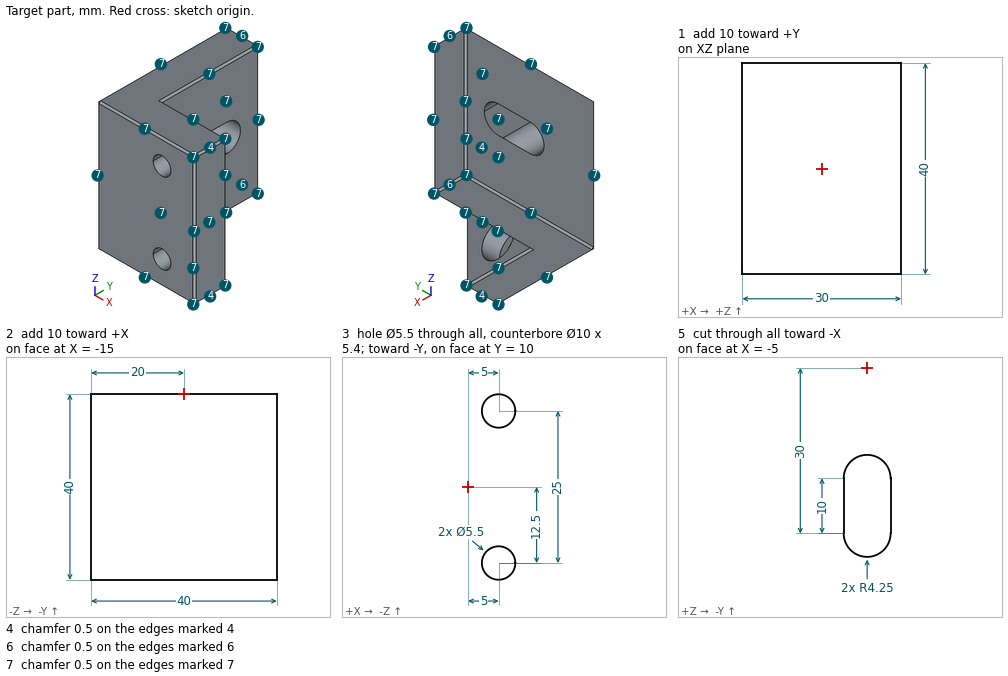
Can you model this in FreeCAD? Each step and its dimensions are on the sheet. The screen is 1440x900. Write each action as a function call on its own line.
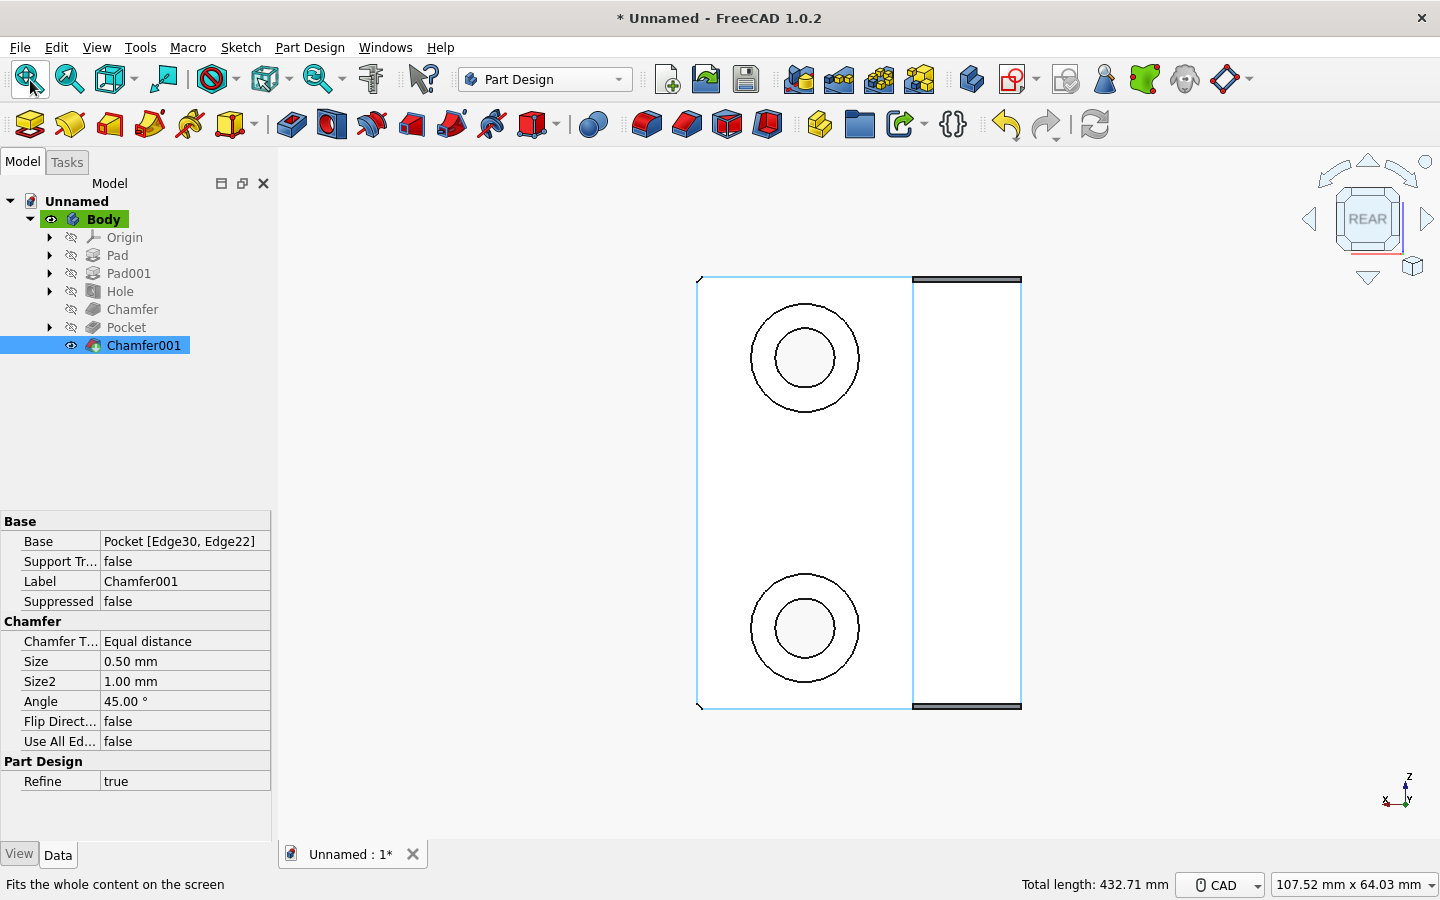
scroll(700, 279, up, 9)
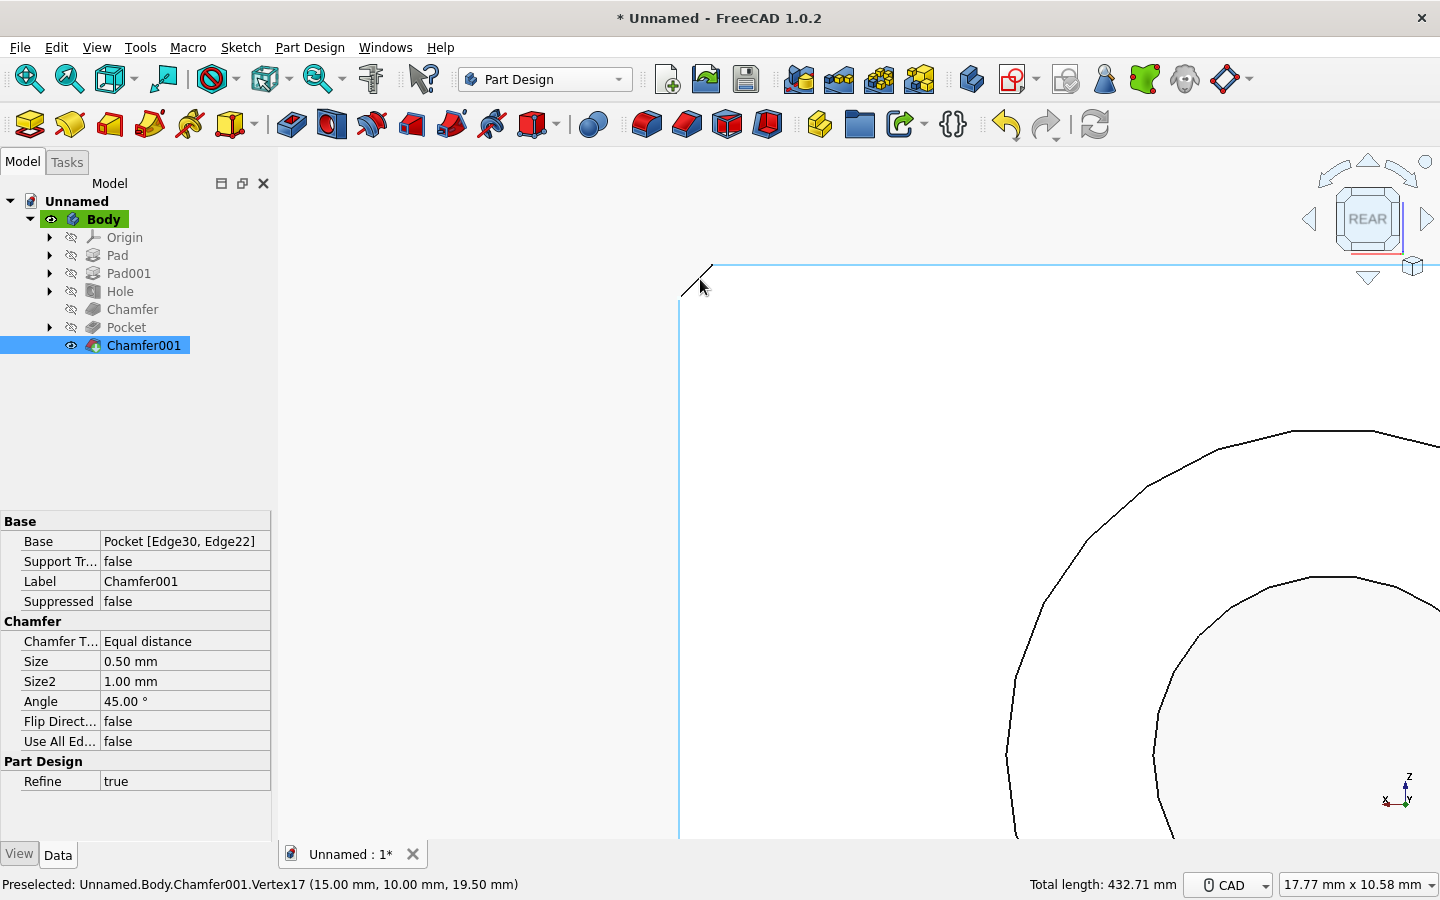
click(30, 80)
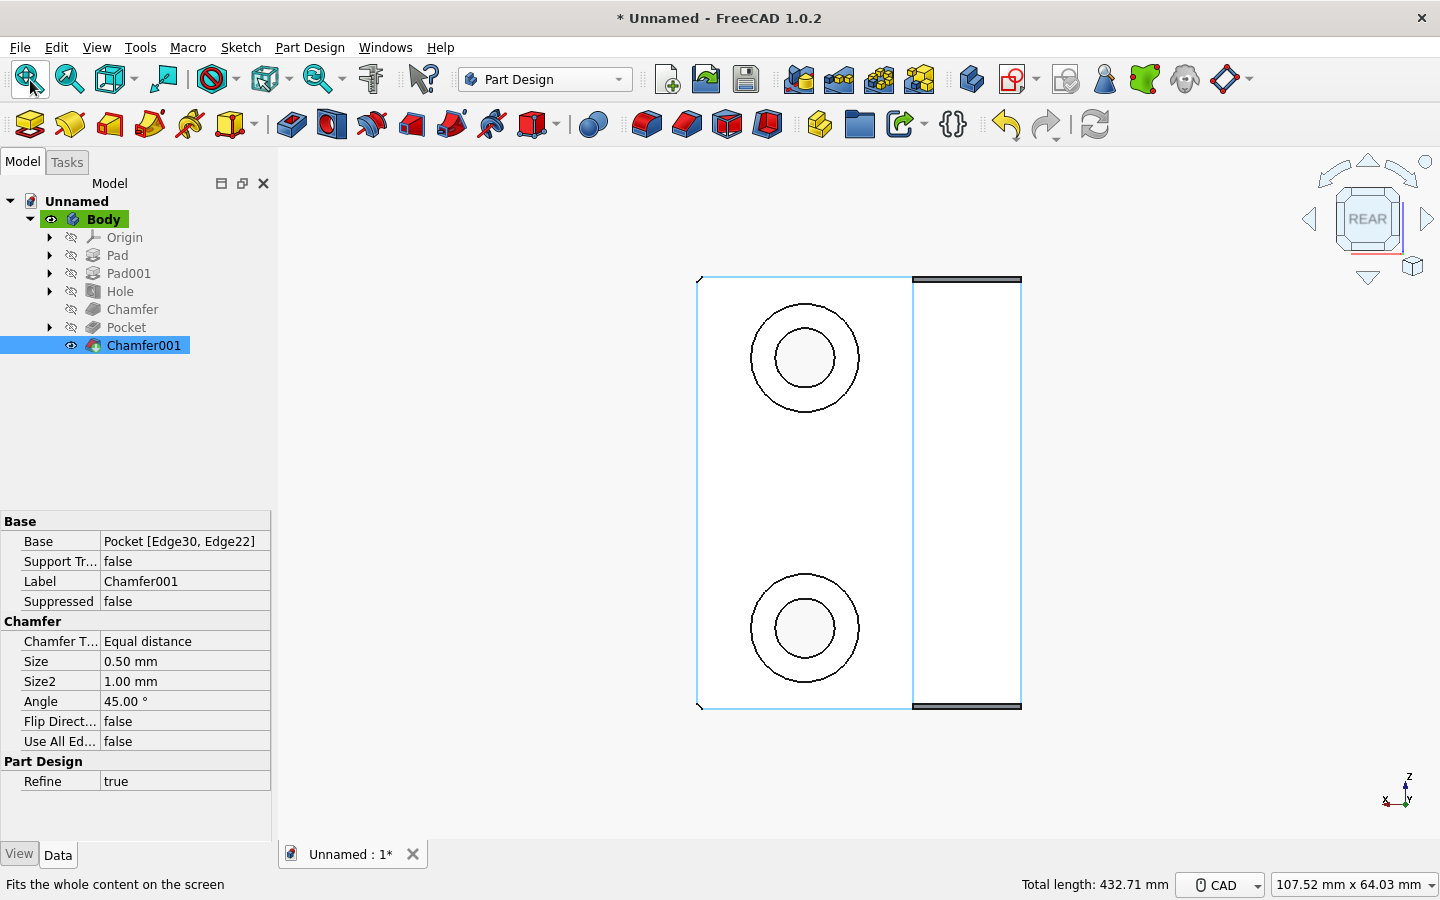
key(6)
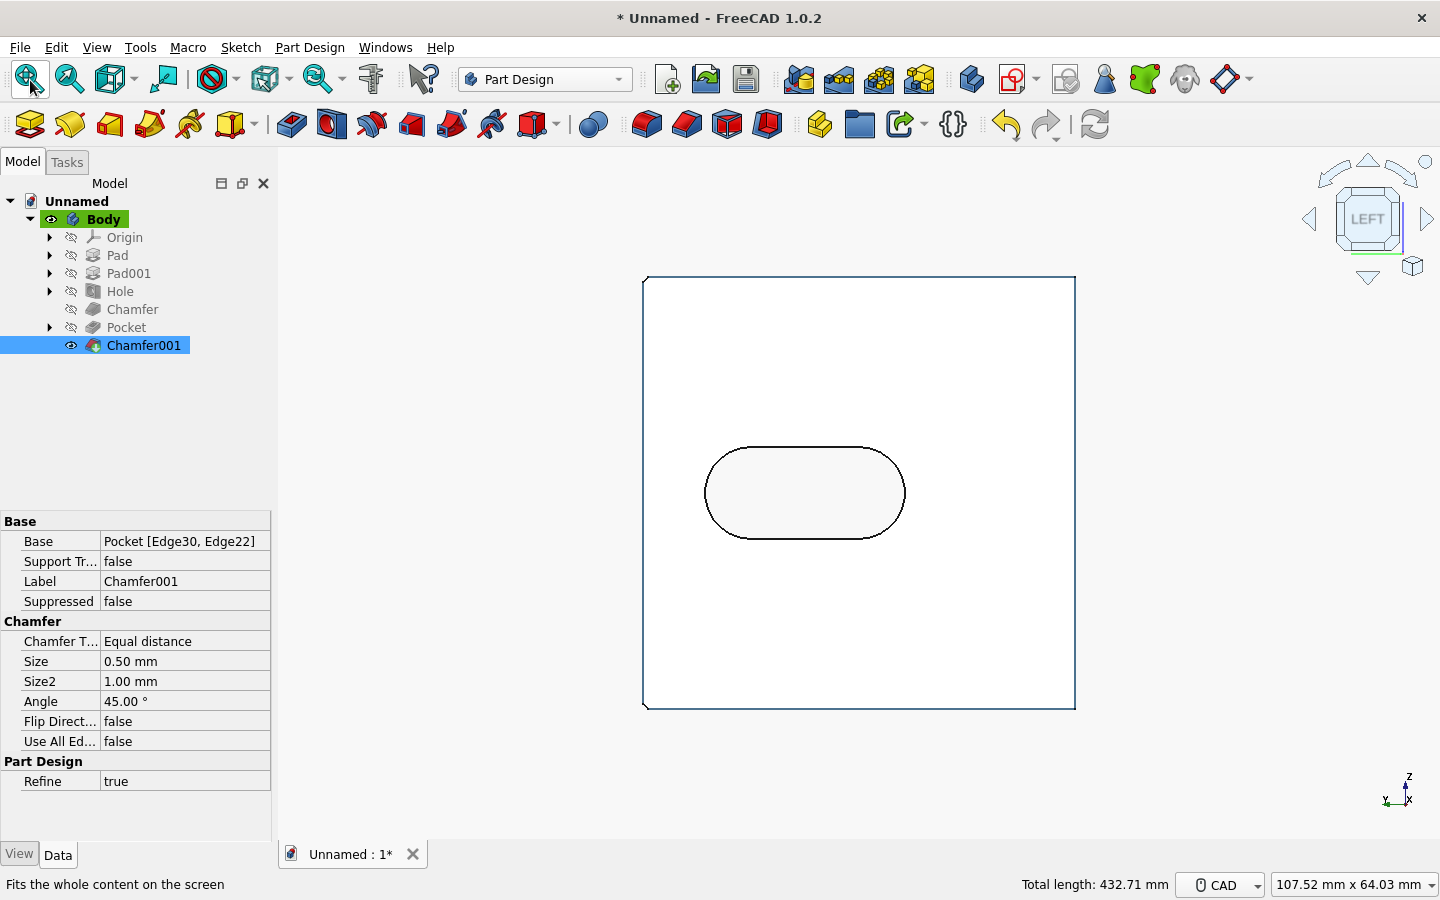
scroll(1075, 279, up, 9)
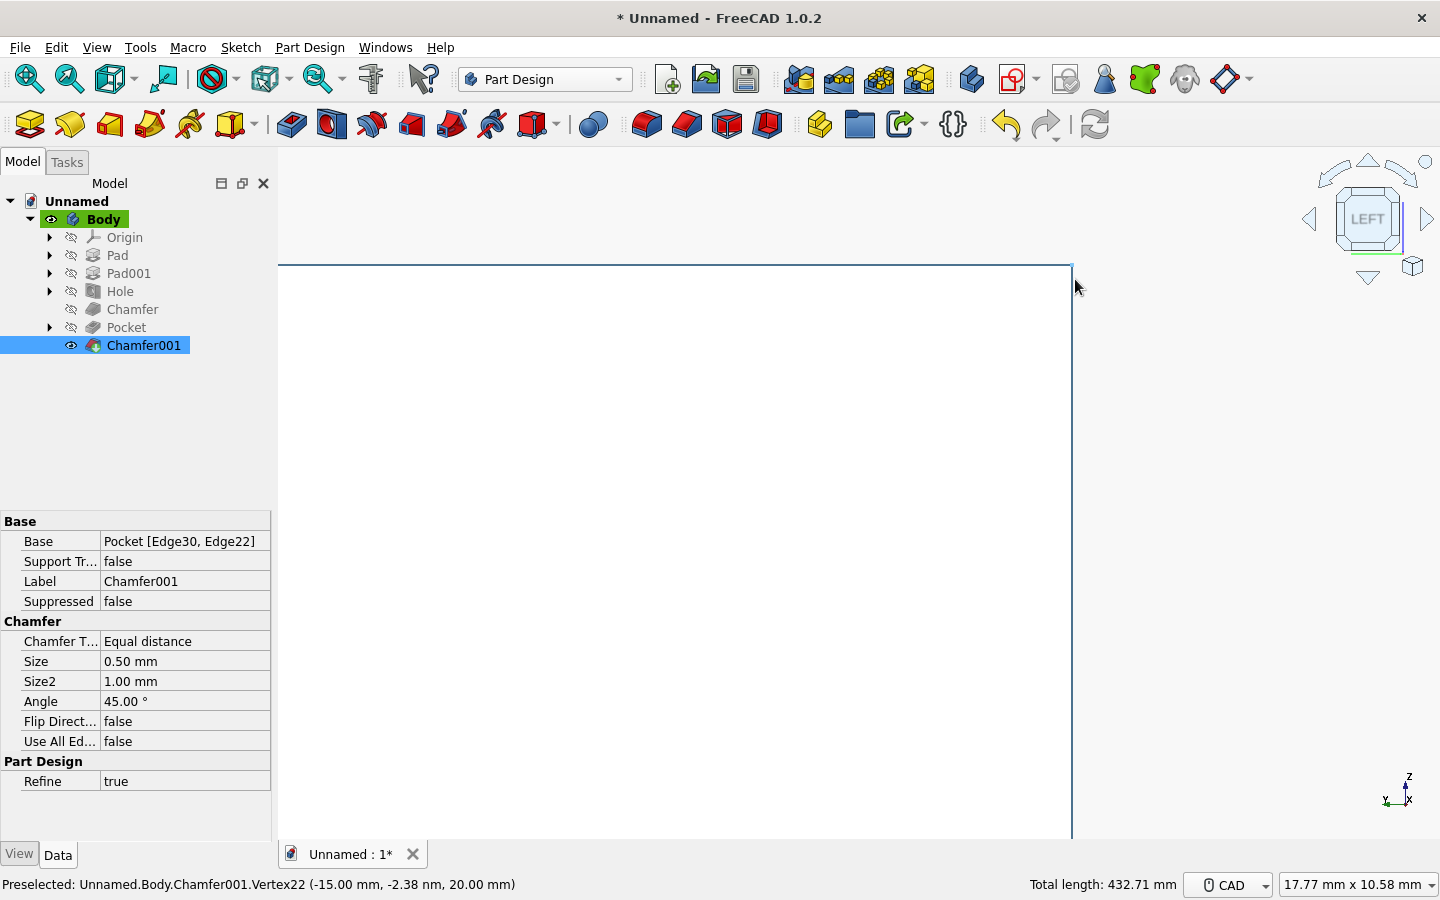
click(30, 80)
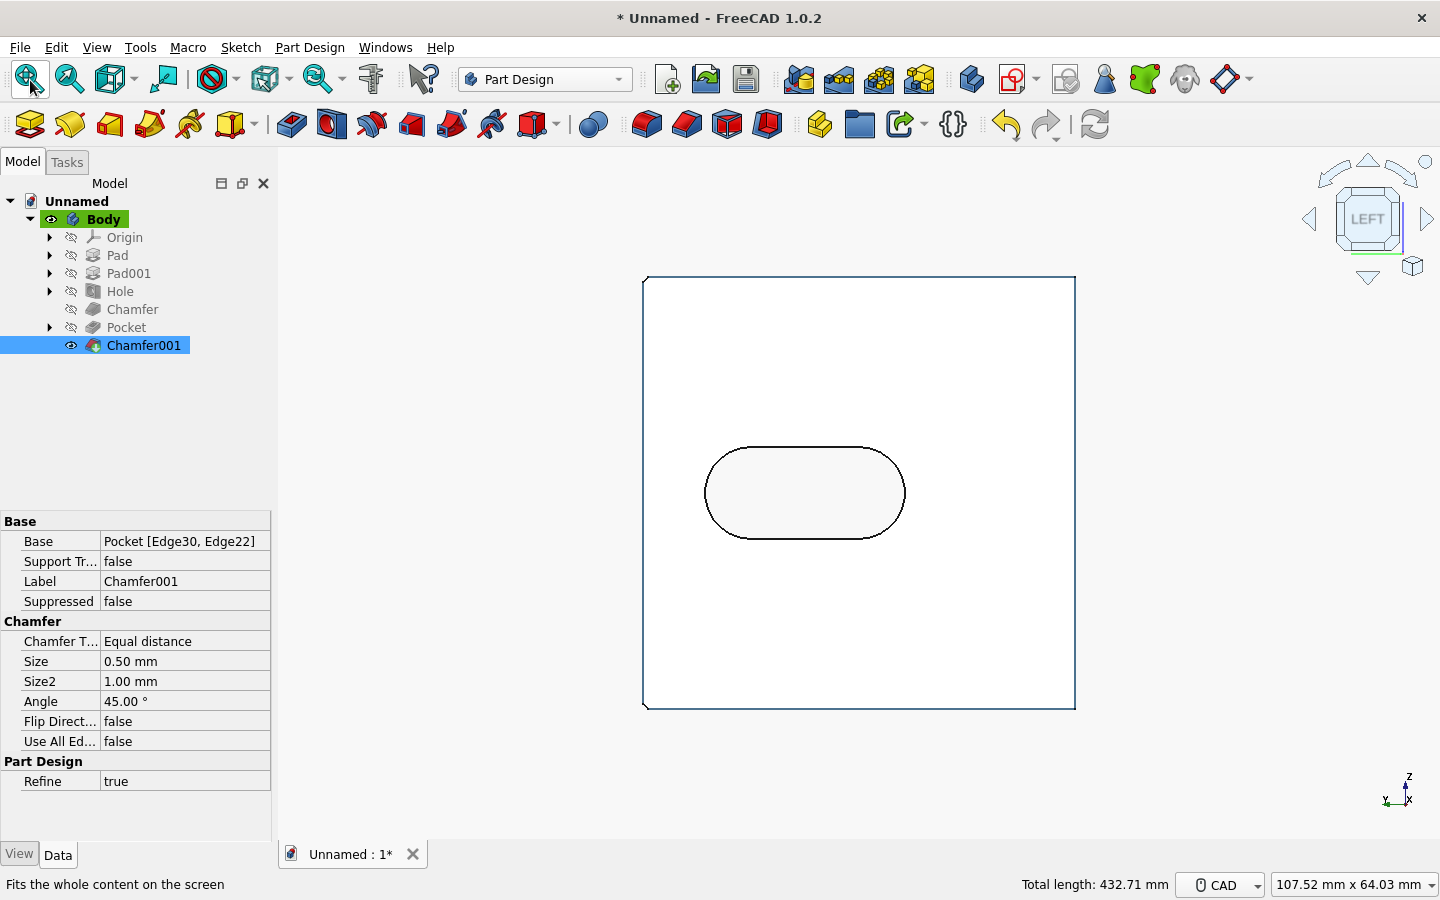
key(v)
key(3)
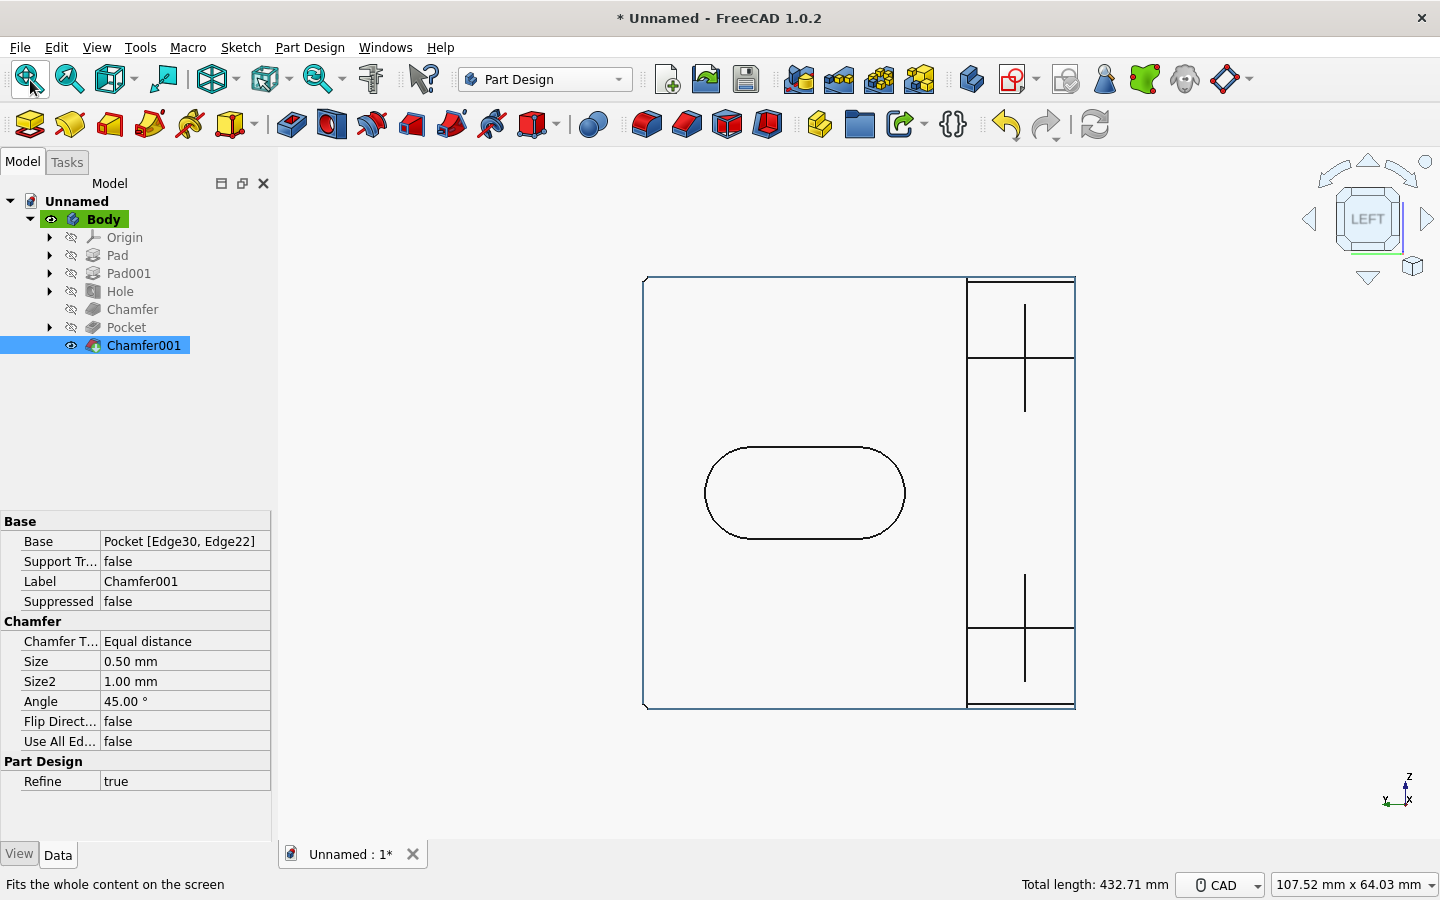
key(0)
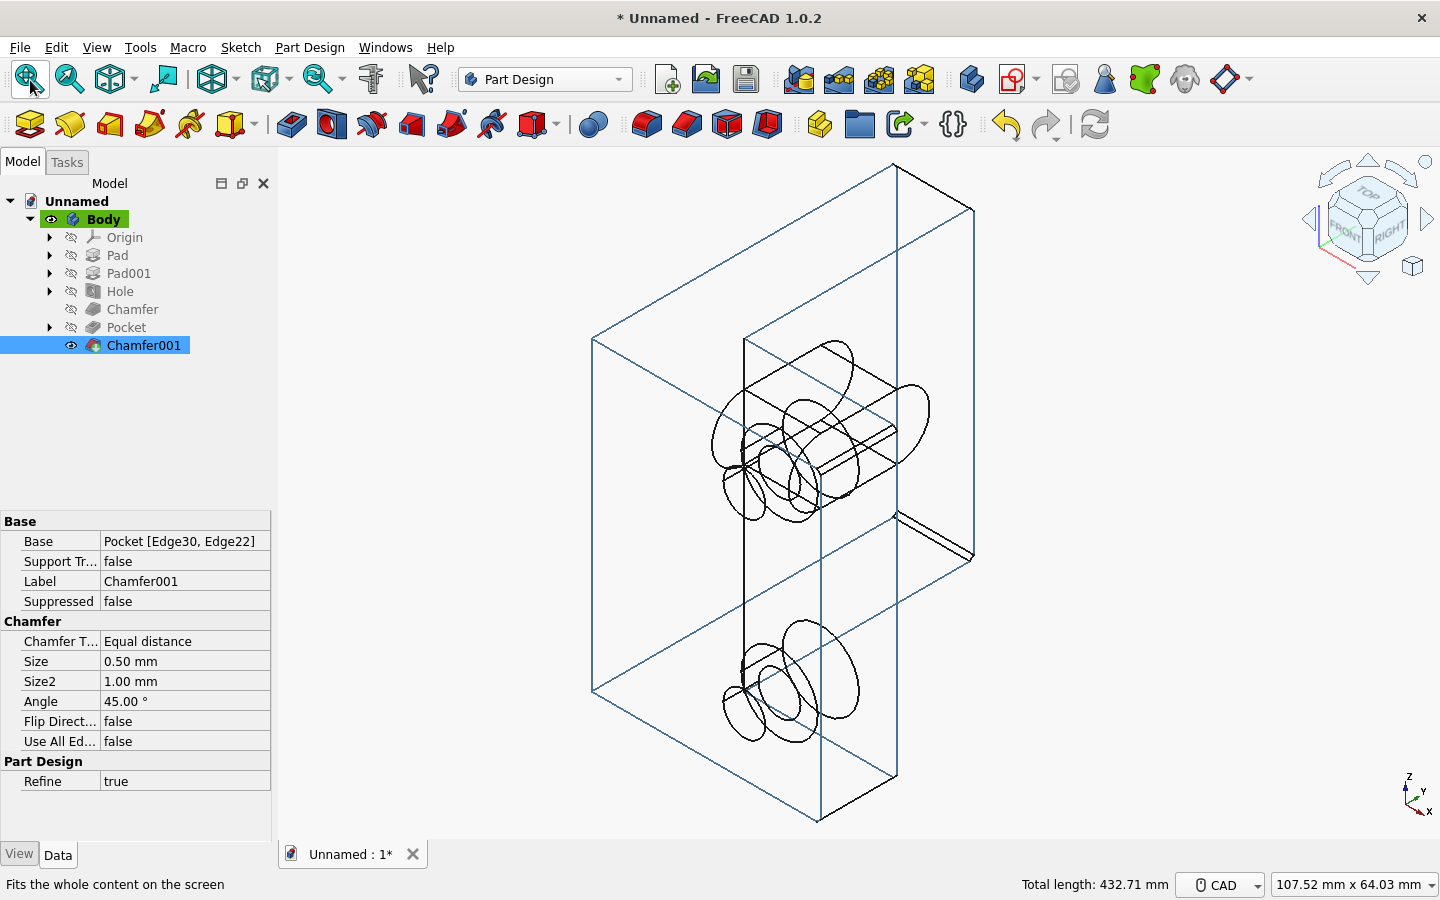
scroll(819, 471, up, 9)